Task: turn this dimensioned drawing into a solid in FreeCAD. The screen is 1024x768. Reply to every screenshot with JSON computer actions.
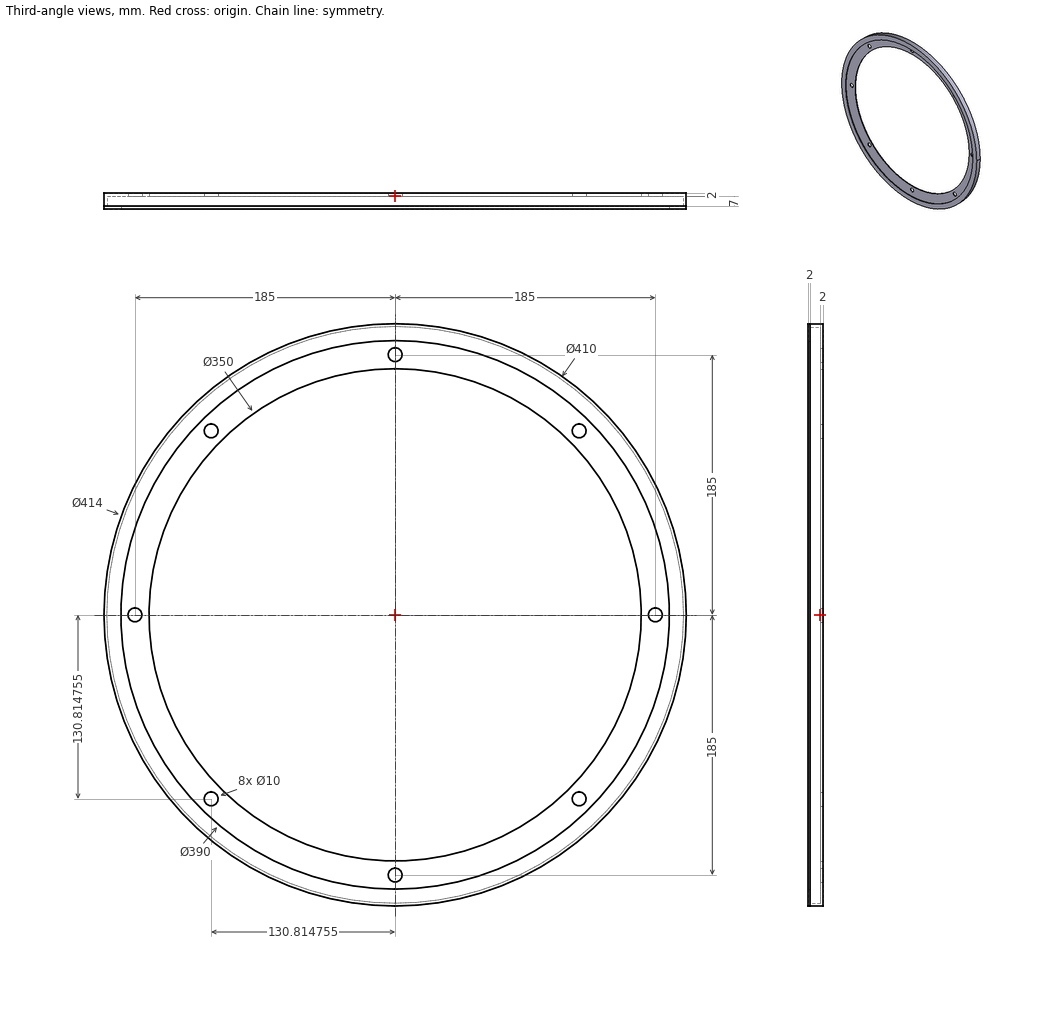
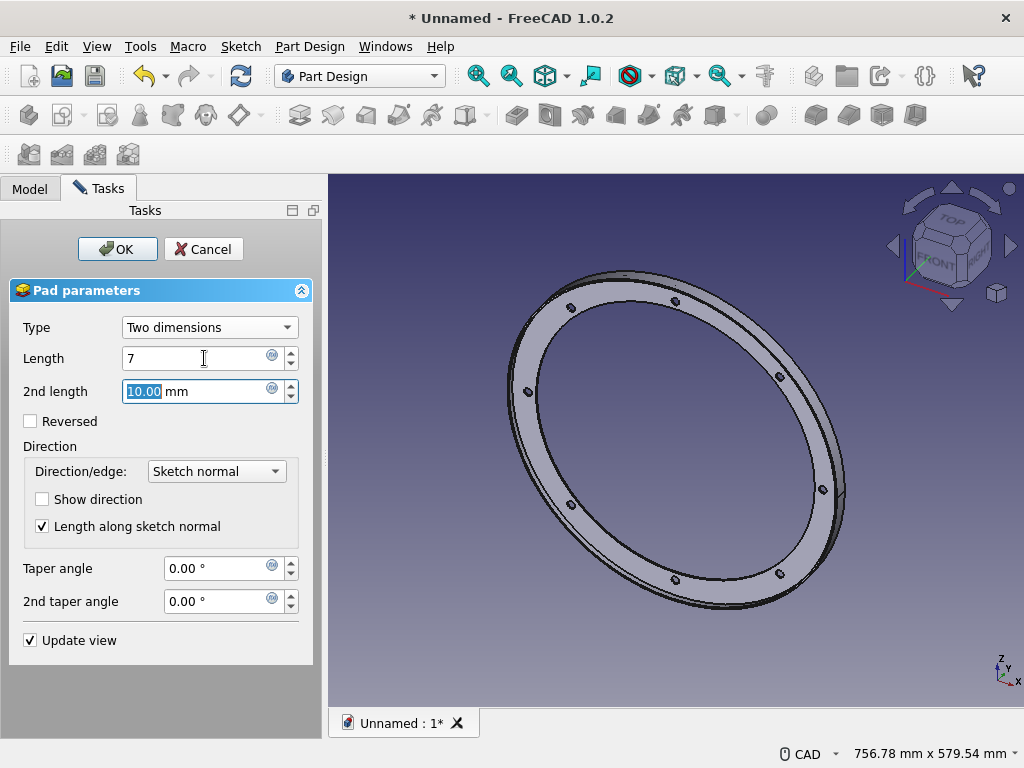
{"action": "type", "text": "2"}
{"action": "key", "text": "Tab"}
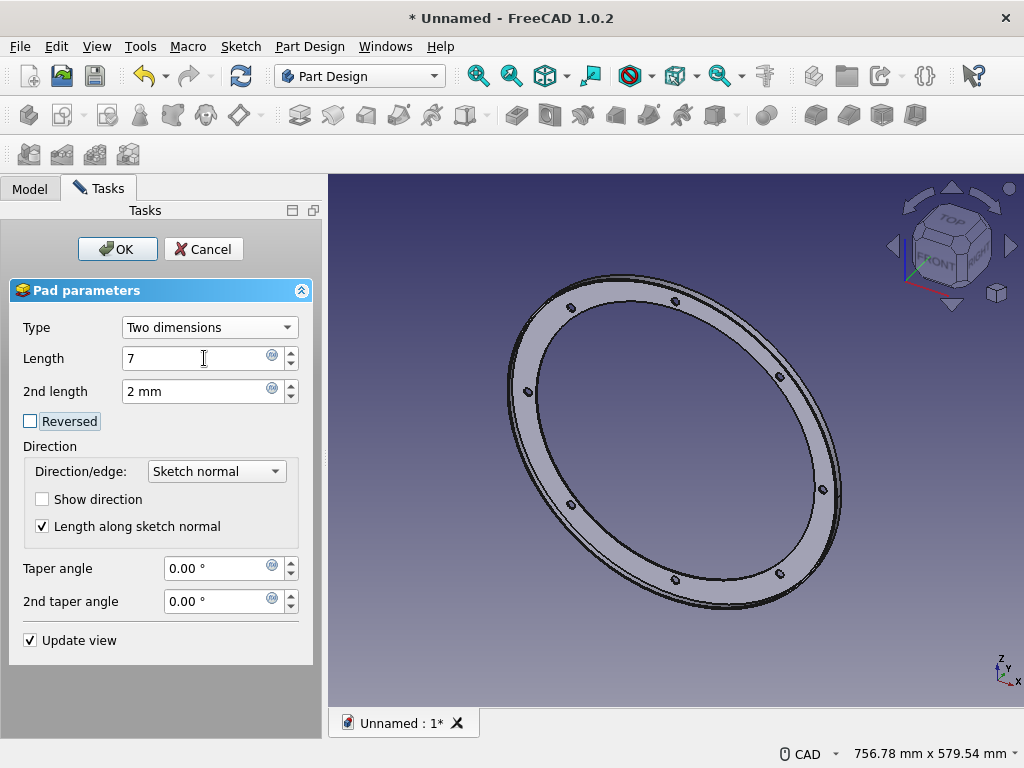
{"action": "left_click", "coordinate": [118, 249]}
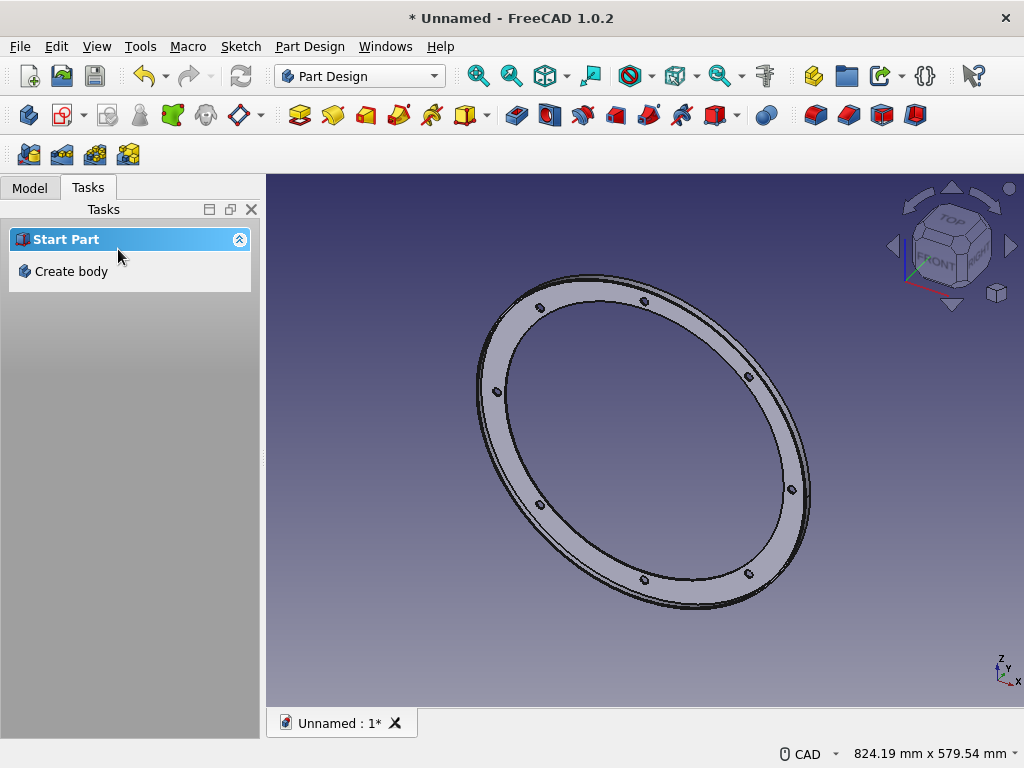
{"action": "left_click", "coordinate": [30, 188]}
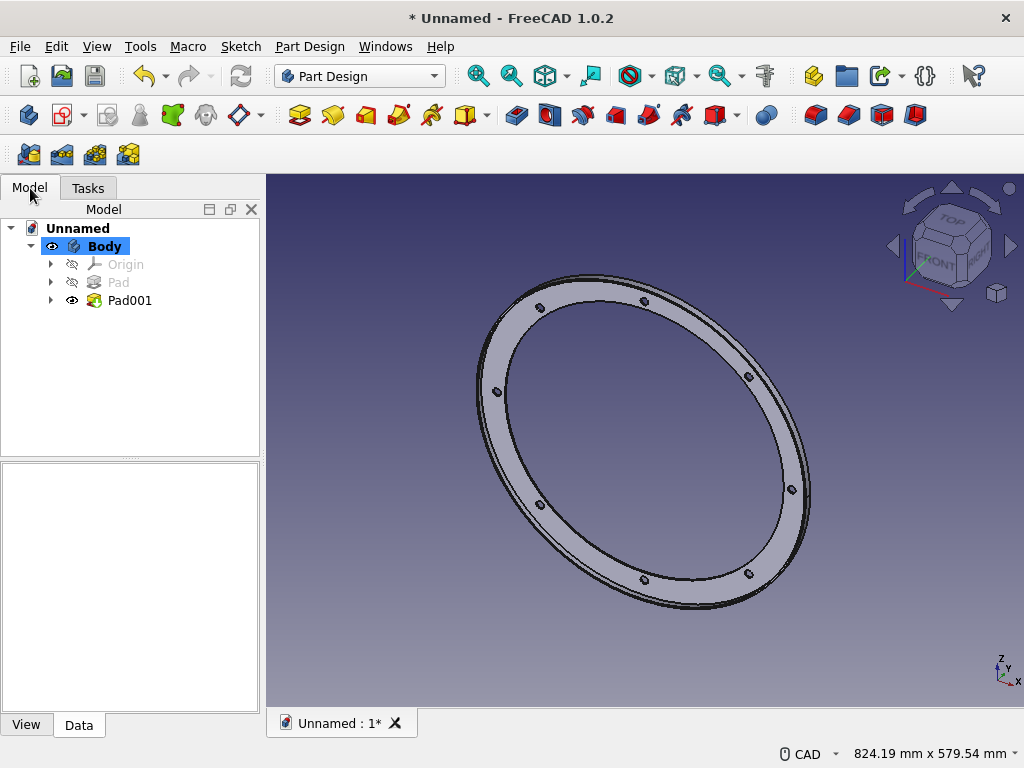
{"action": "left_click", "coordinate": [51, 264]}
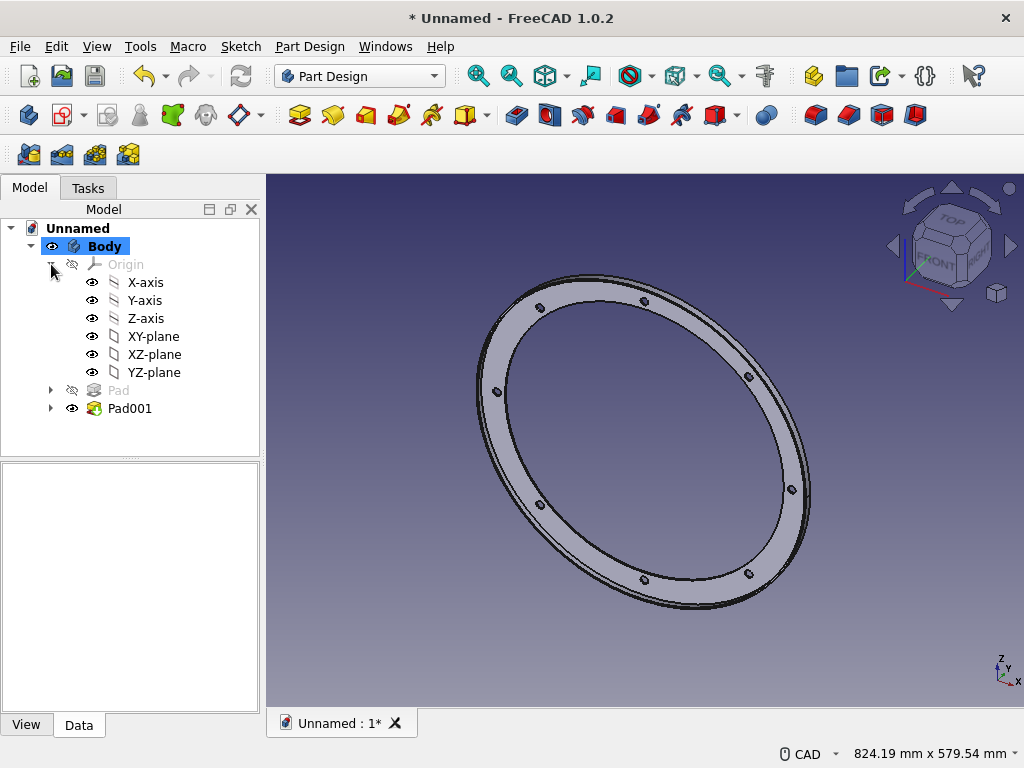
{"action": "left_click", "coordinate": [137, 354]}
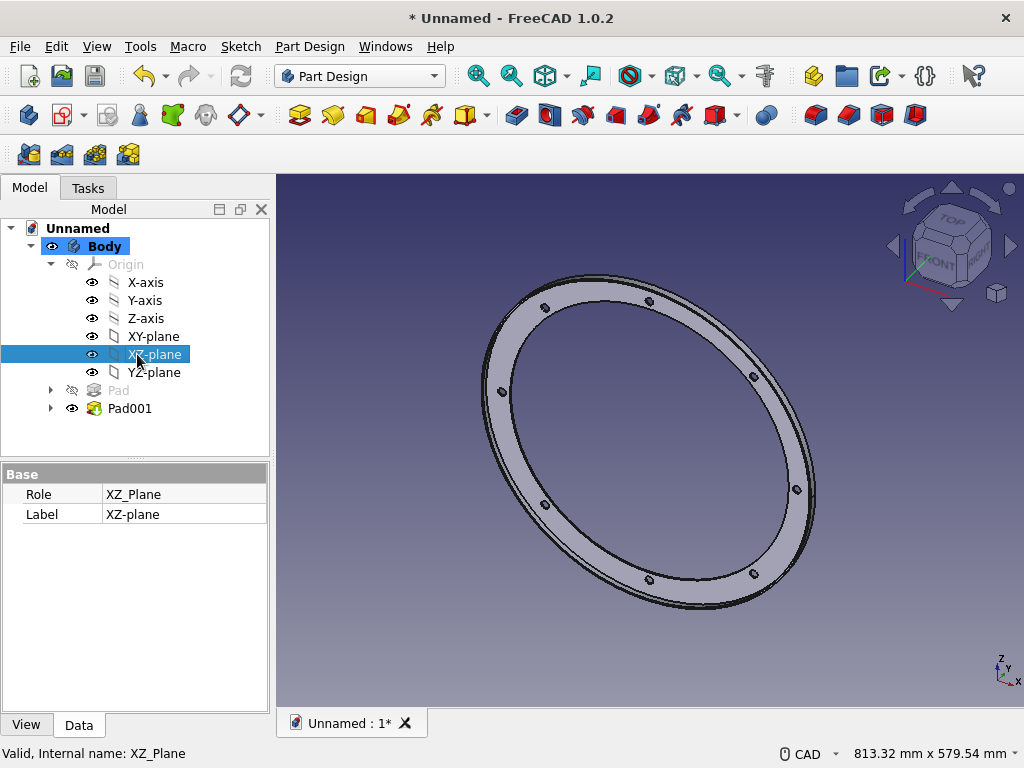
{"action": "left_click", "coordinate": [238, 116]}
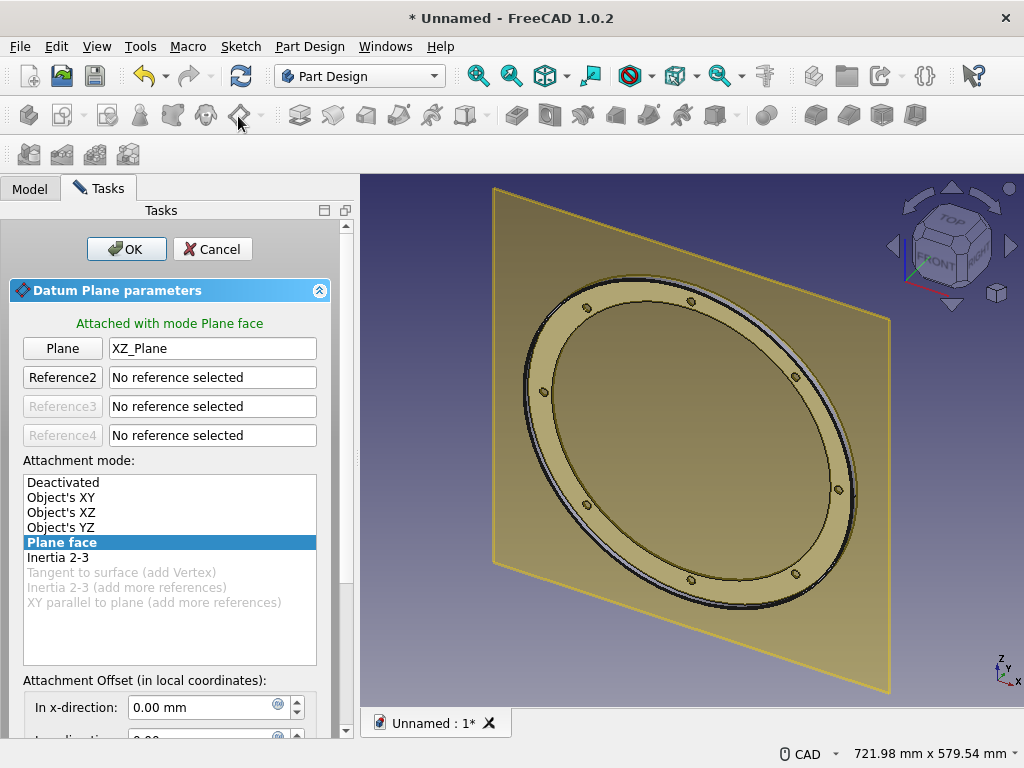
{"action": "scroll", "coordinate": [346, 479], "scroll_direction": "down", "scroll_amount": 2}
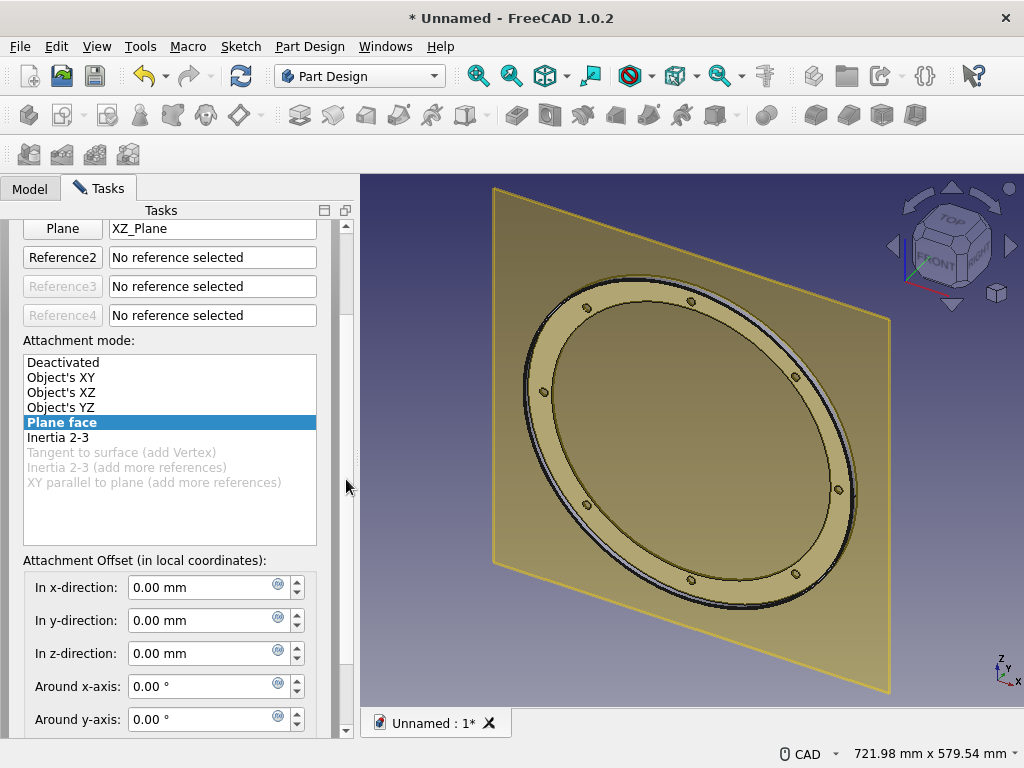
{"action": "triple_click", "coordinate": [210, 654]}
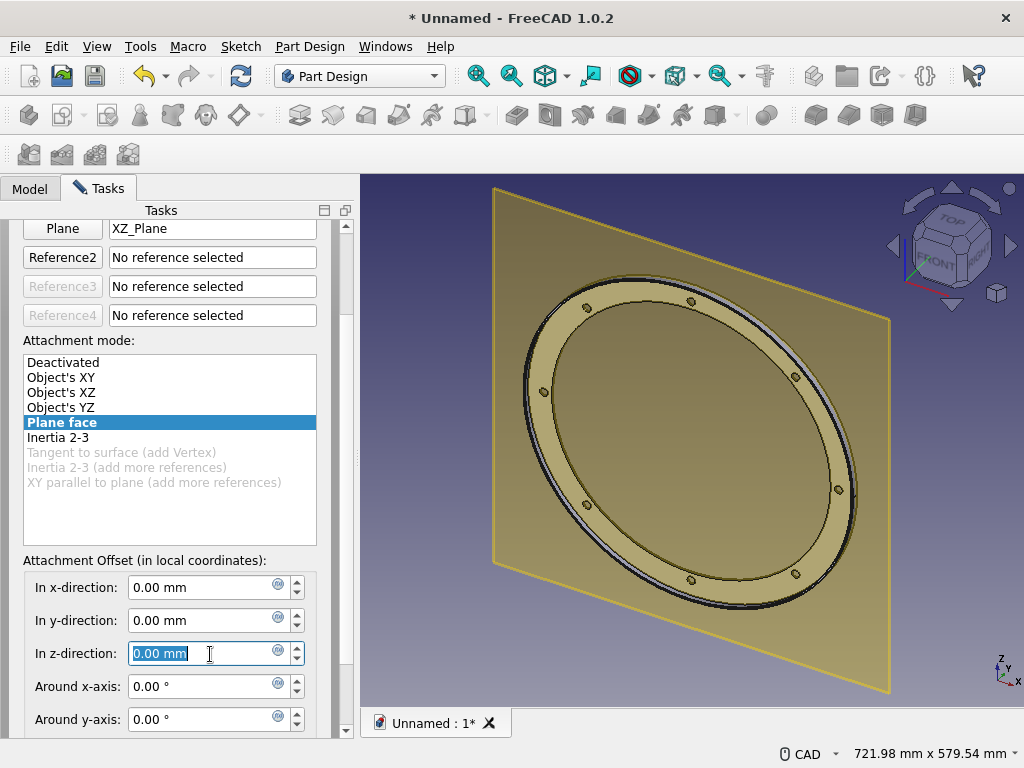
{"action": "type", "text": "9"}
{"action": "key", "text": "Tab"}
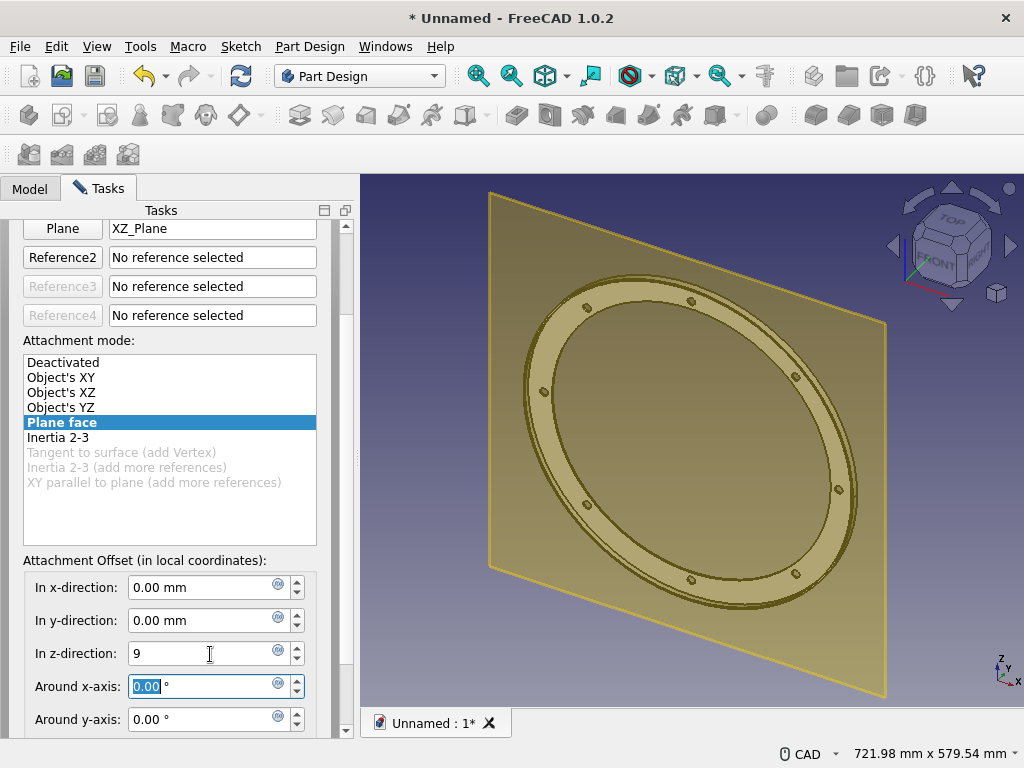
{"action": "scroll", "coordinate": [346, 479], "scroll_direction": "up", "scroll_amount": 3}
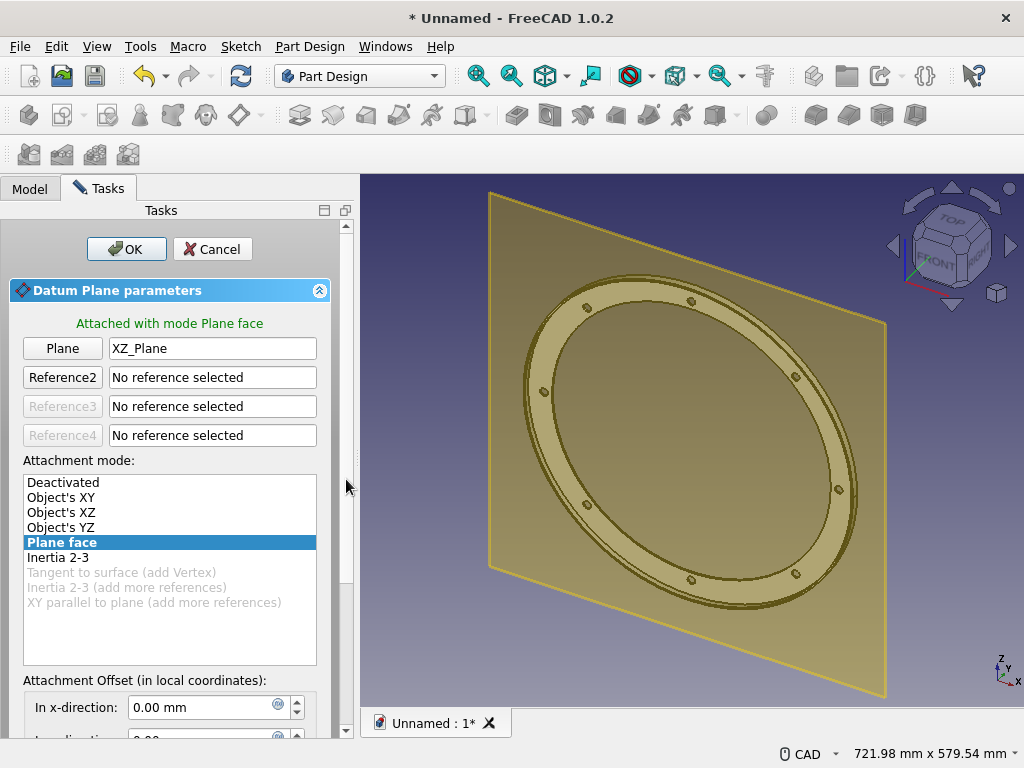
{"action": "left_click", "coordinate": [127, 249]}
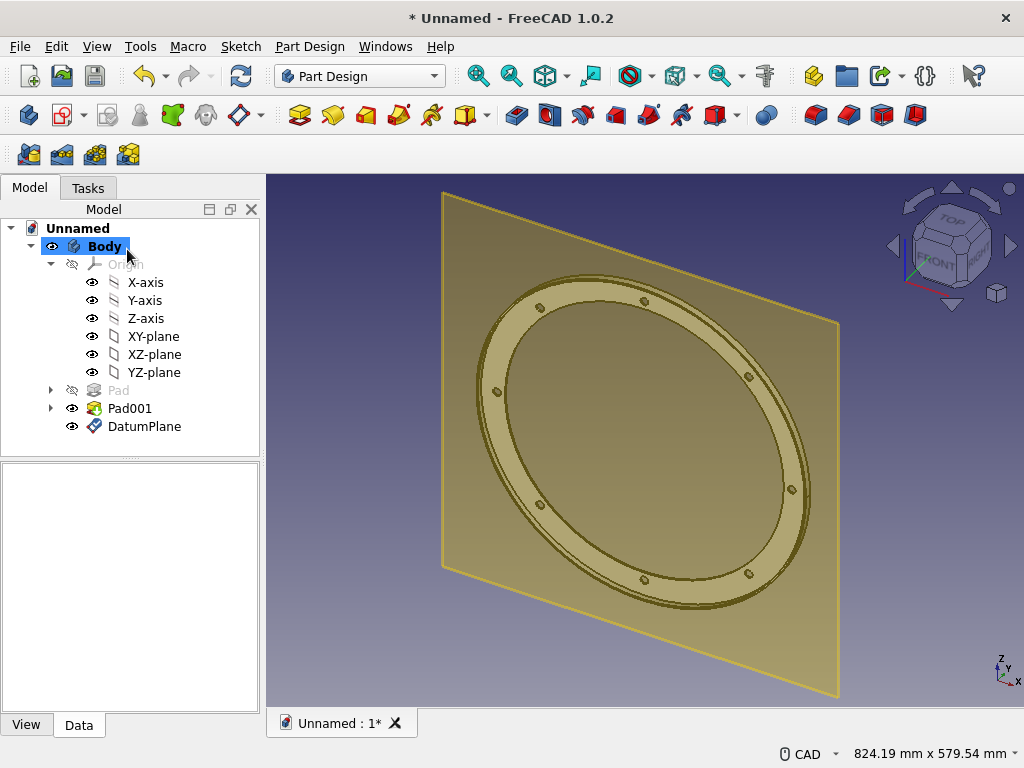
{"action": "left_click", "coordinate": [117, 426]}